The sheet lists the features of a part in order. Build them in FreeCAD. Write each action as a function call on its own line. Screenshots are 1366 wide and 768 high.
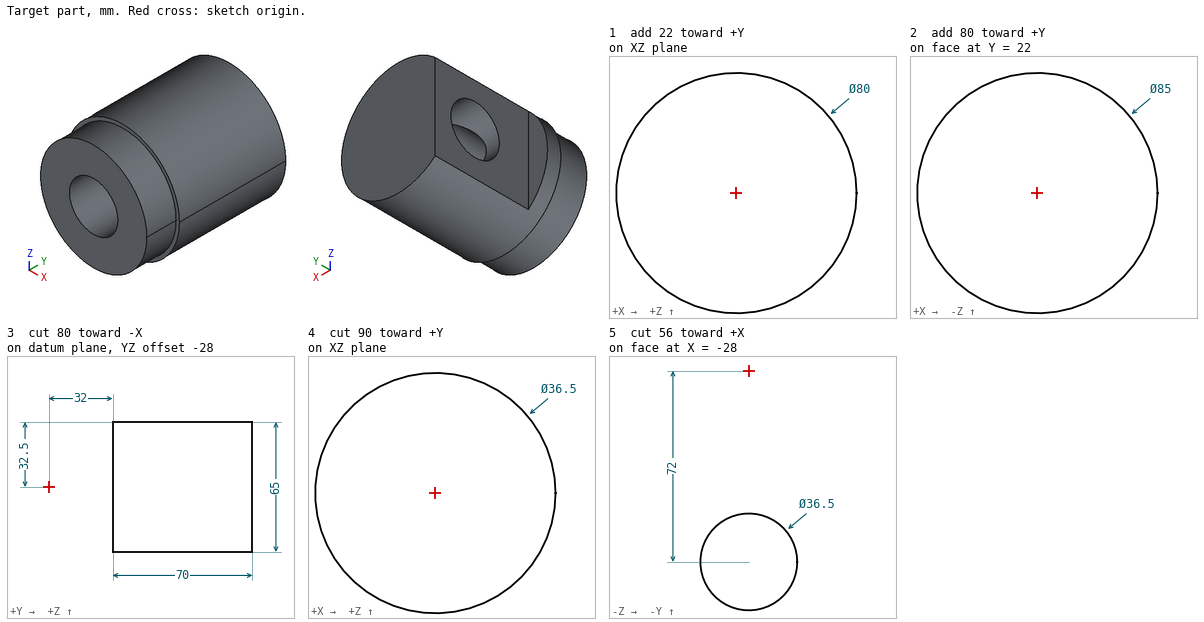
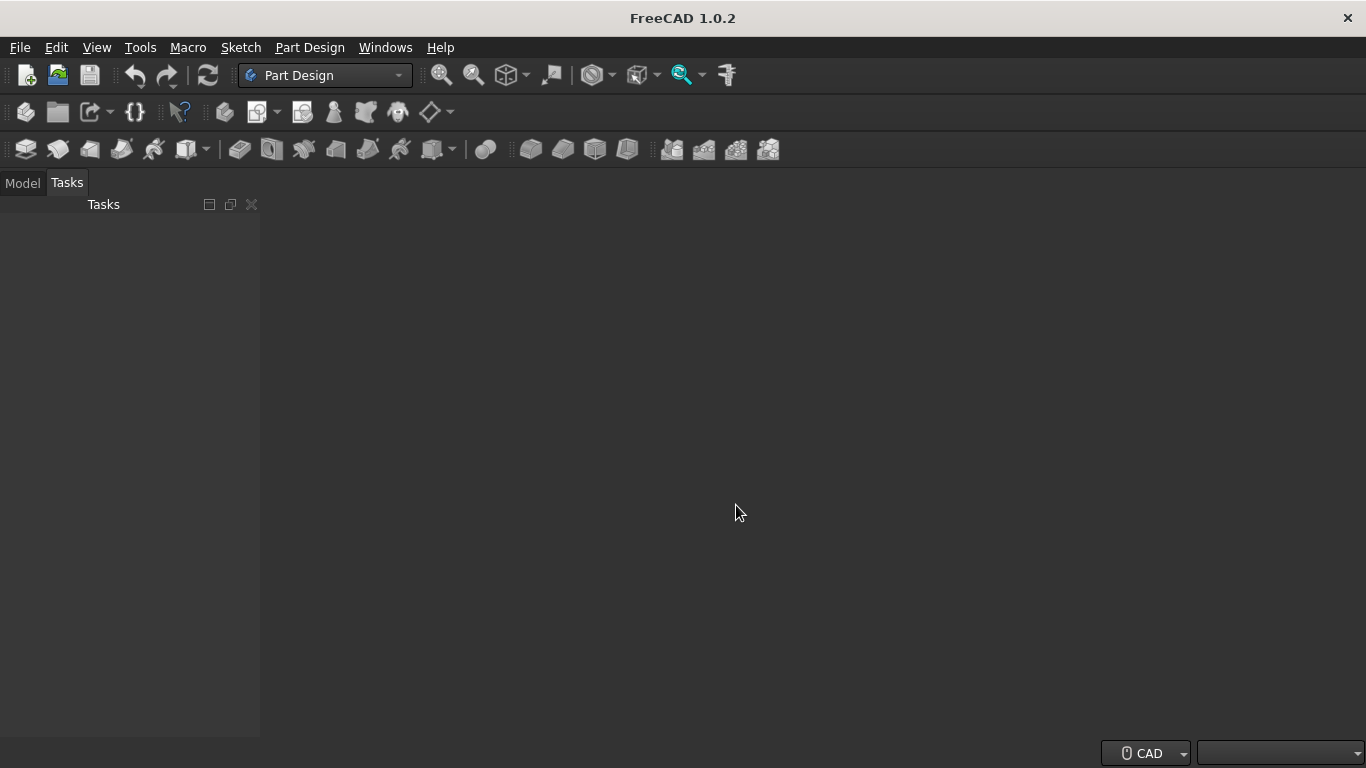
click(26, 76)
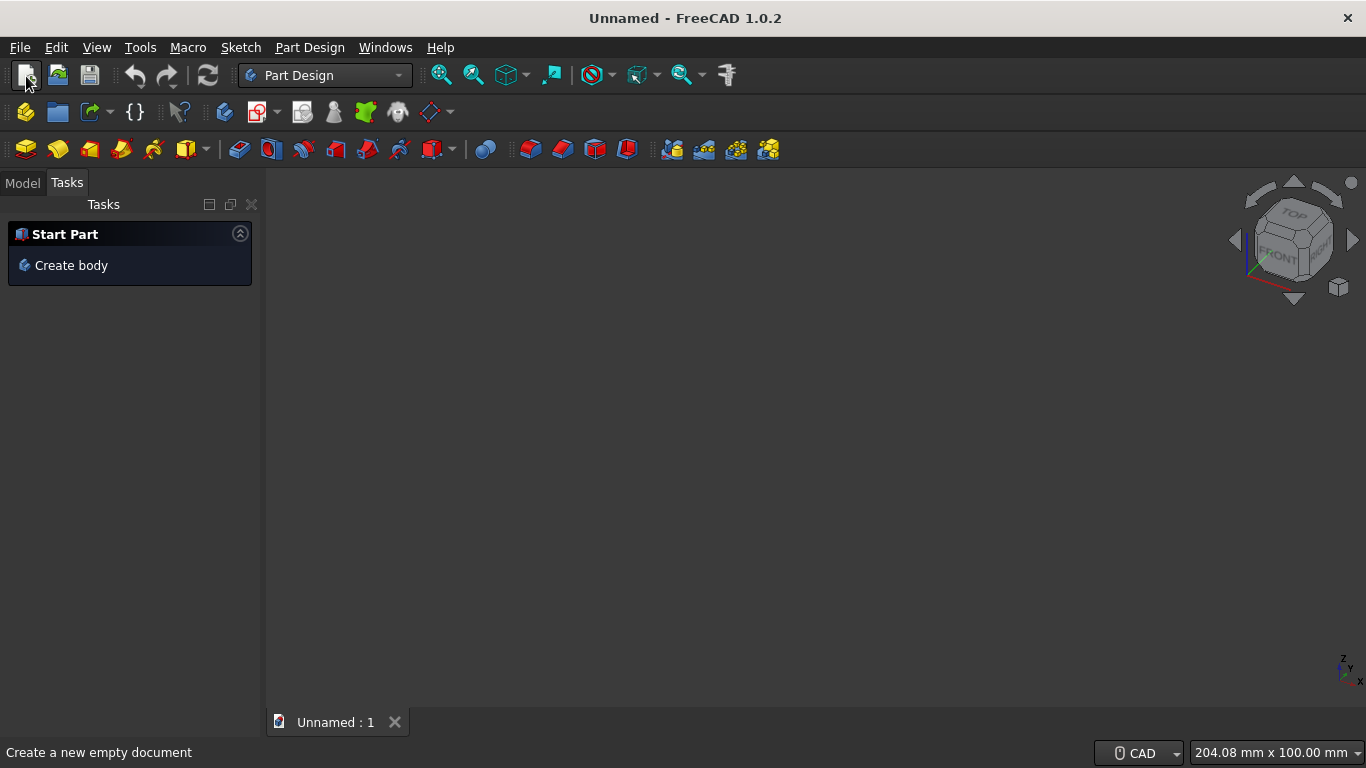
click(258, 112)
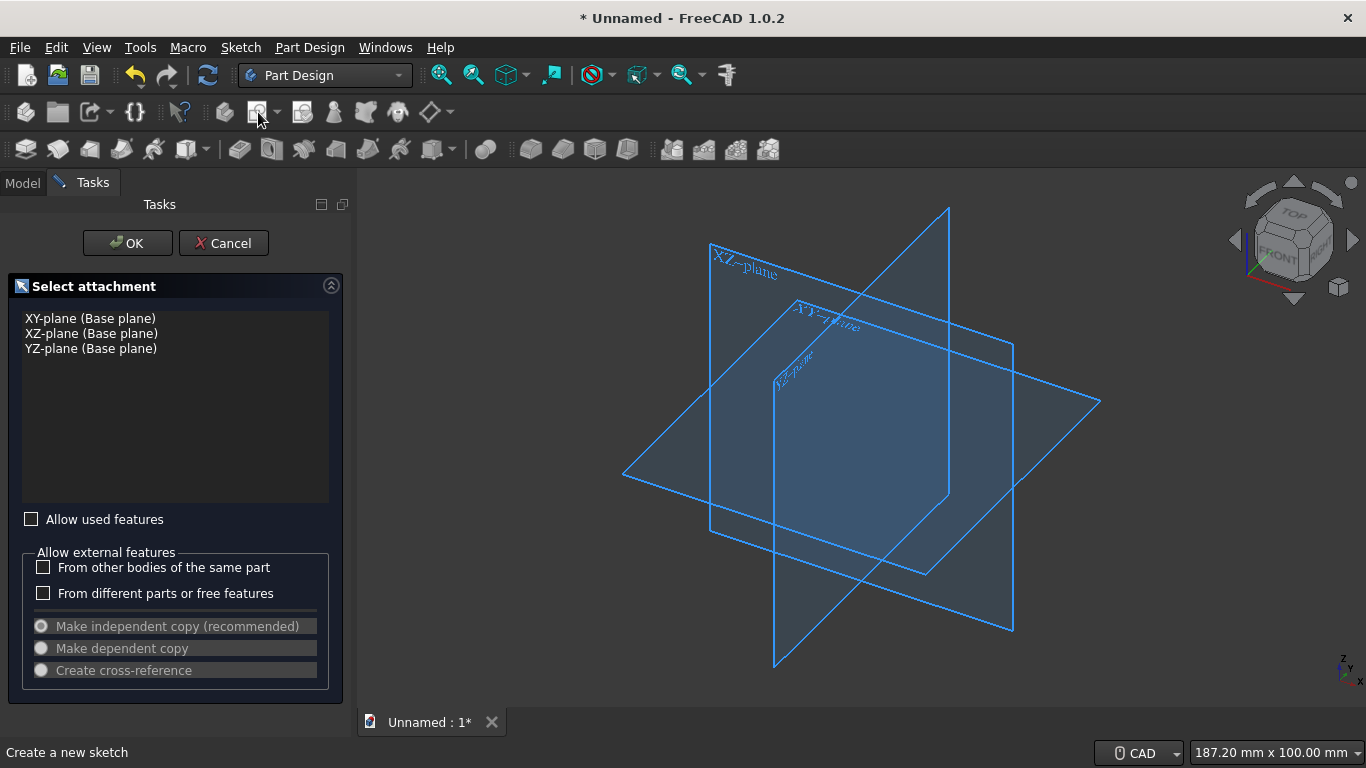
click(82, 334)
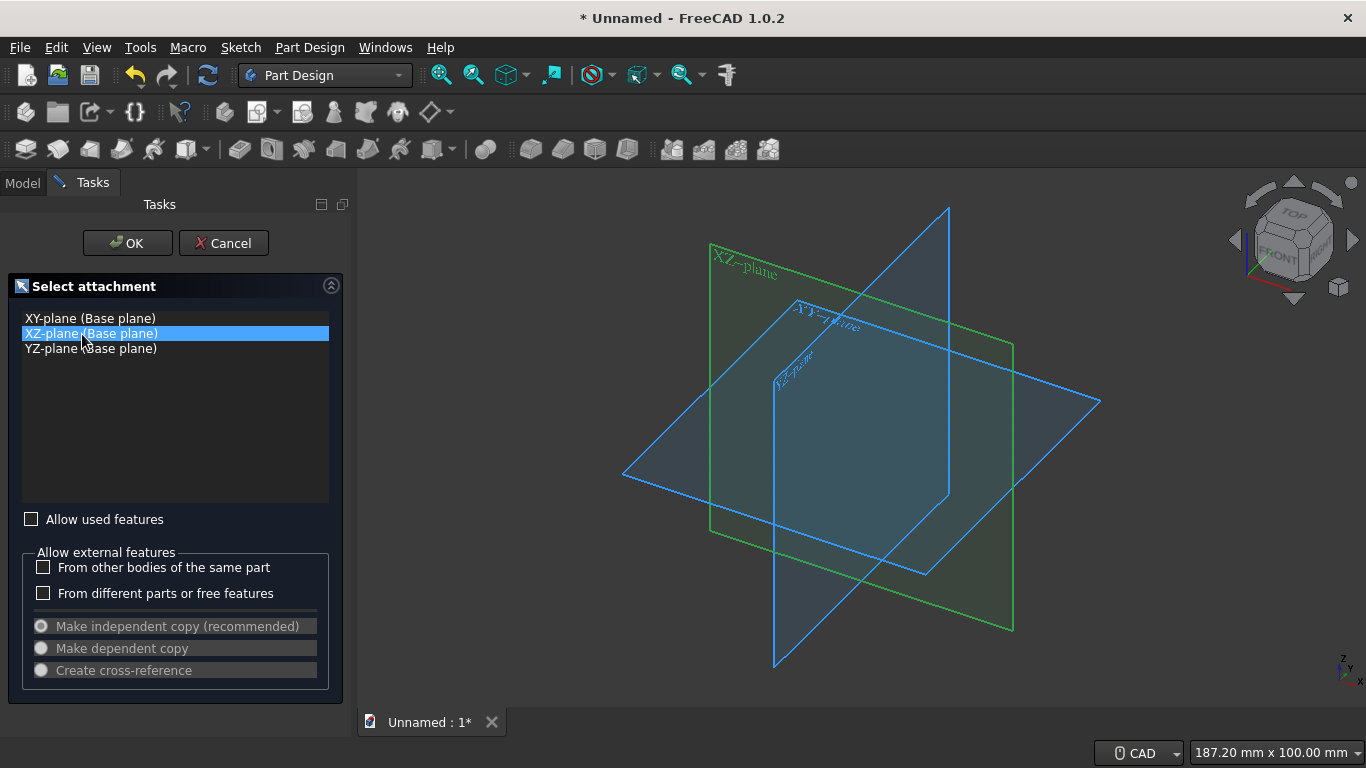
click(128, 243)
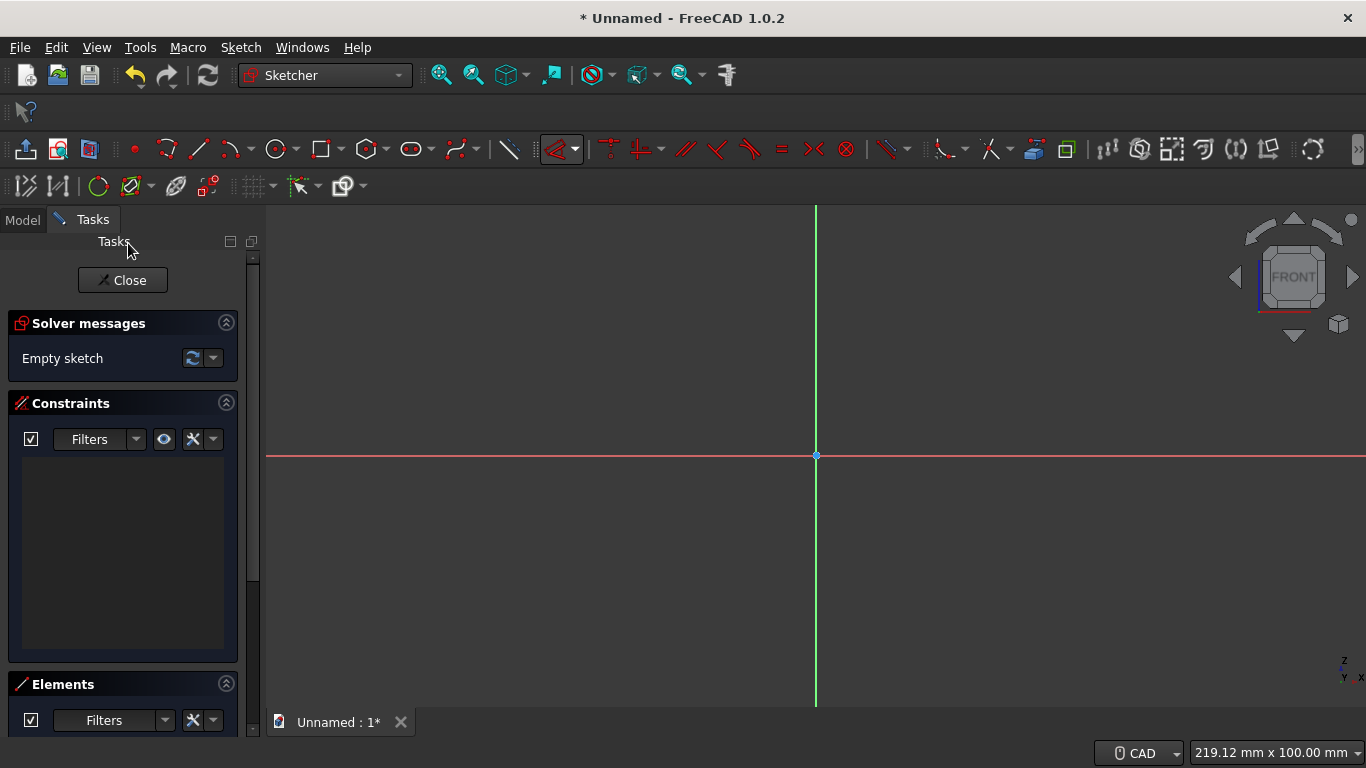
scroll(438, 456, down, 1)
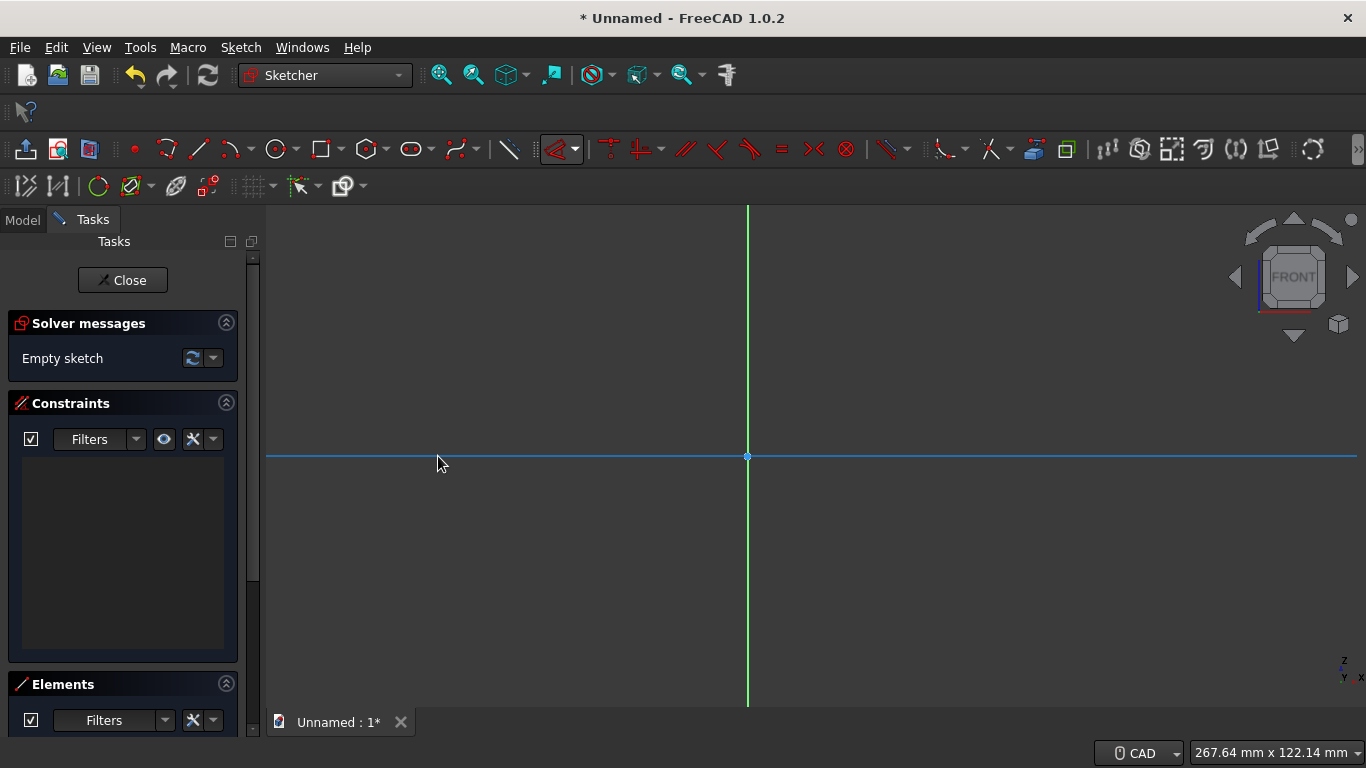
click(276, 150)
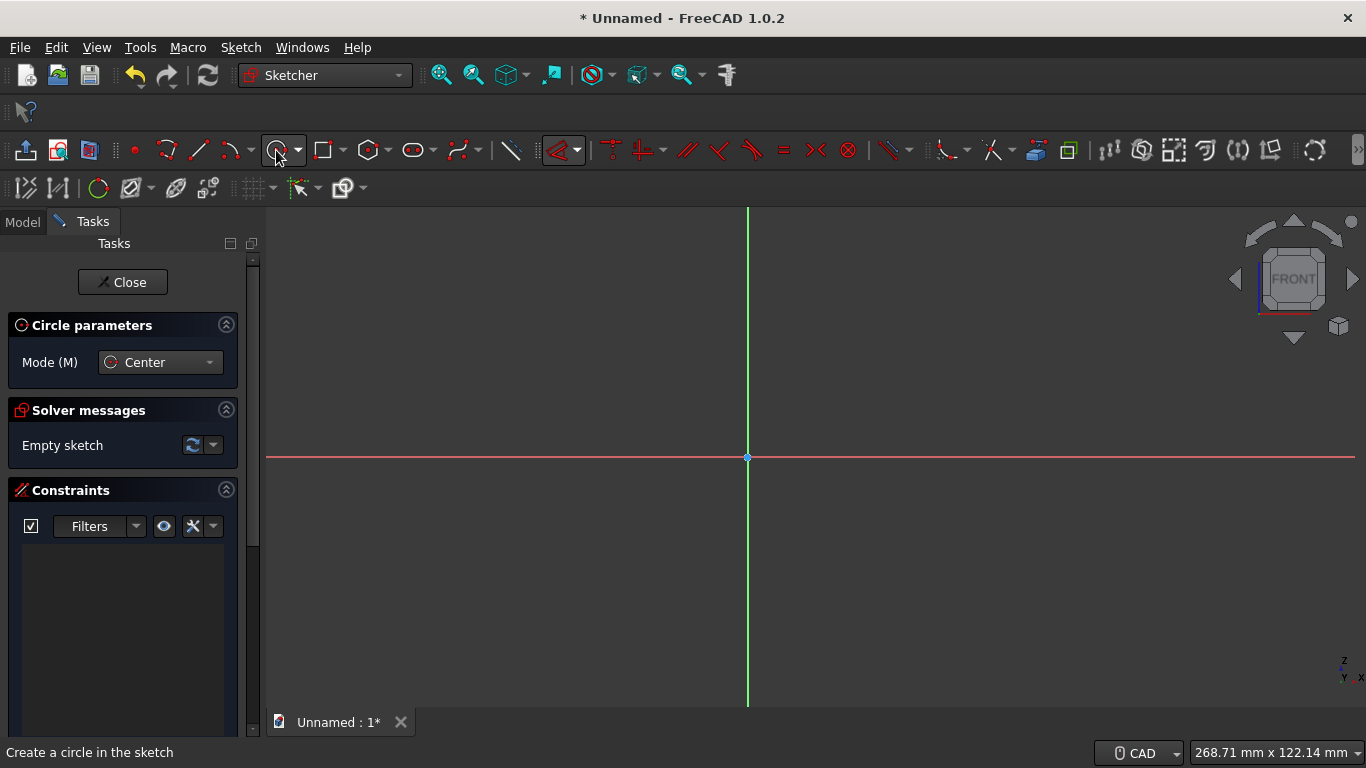
click(748, 457)
move(864, 341)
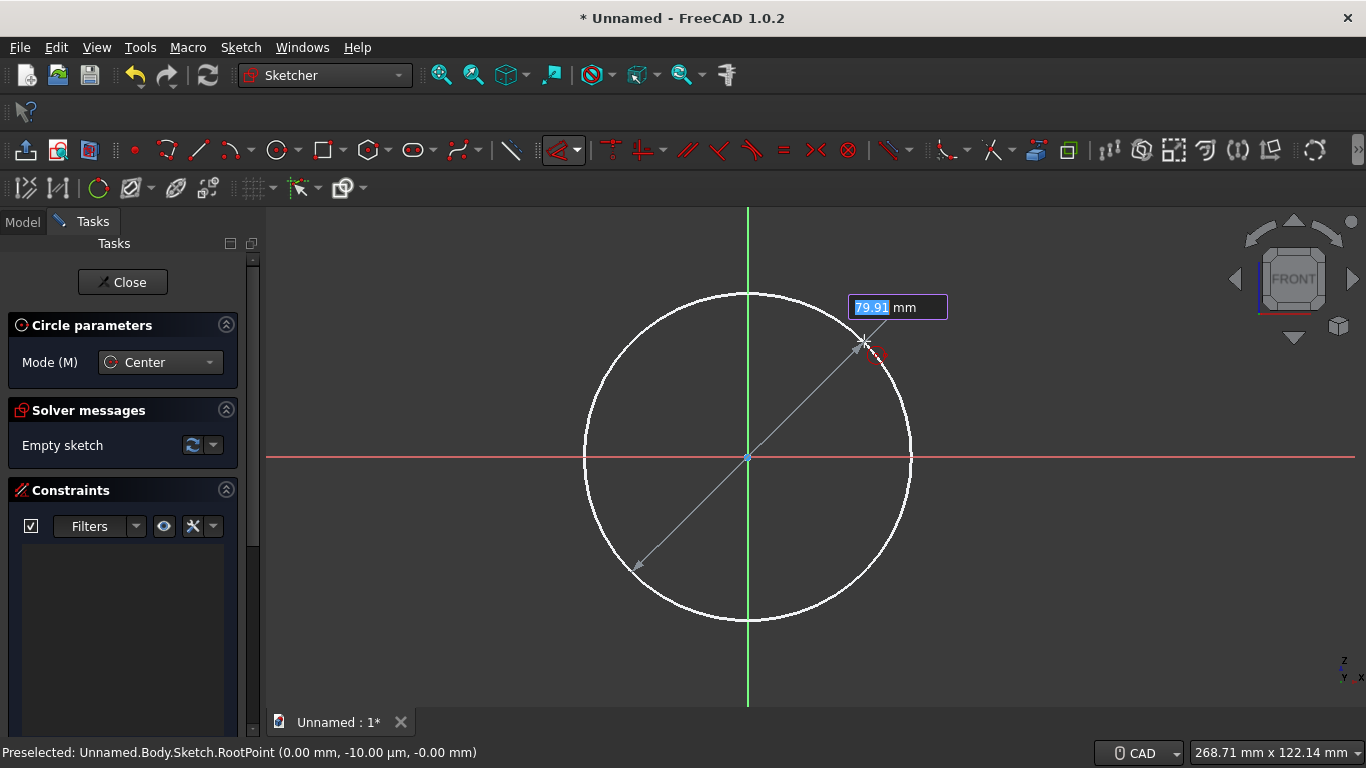
text(80)
key(Return)
key(Escape)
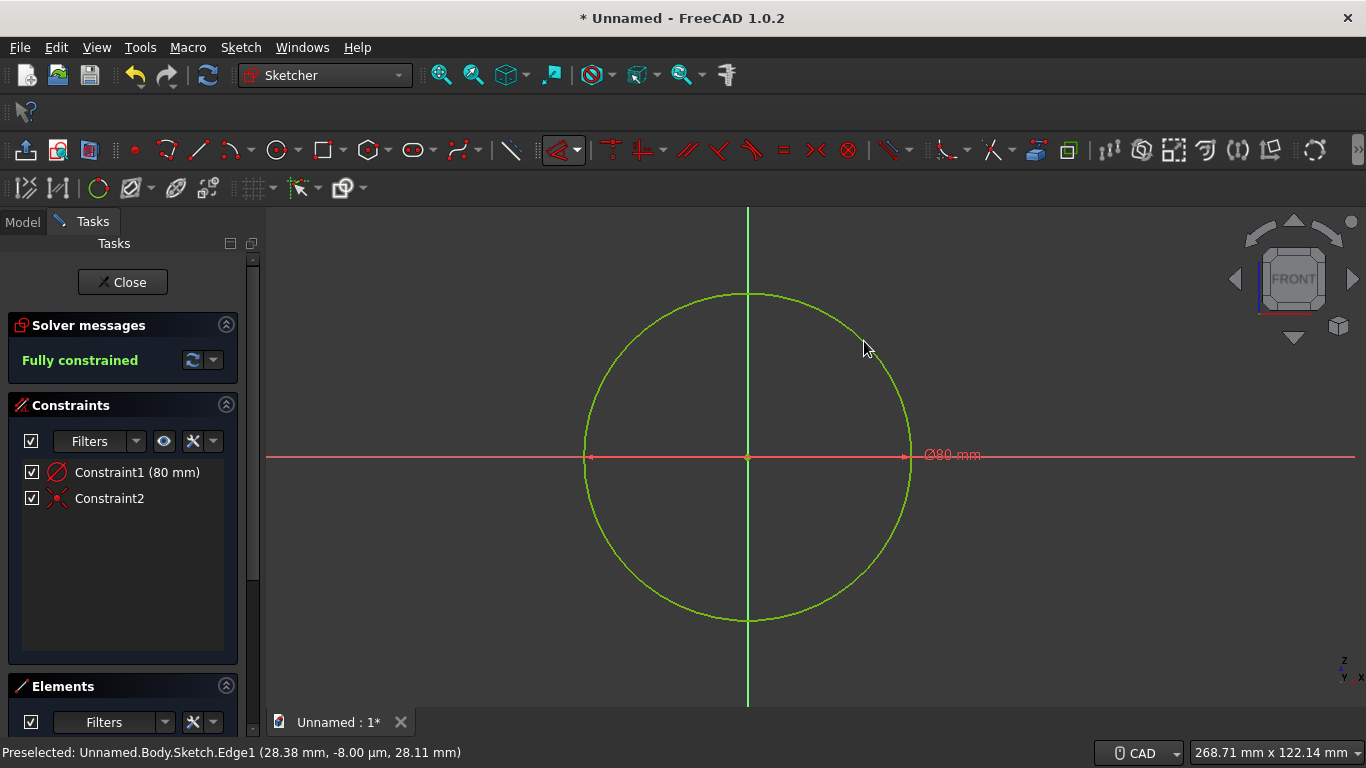
click(123, 282)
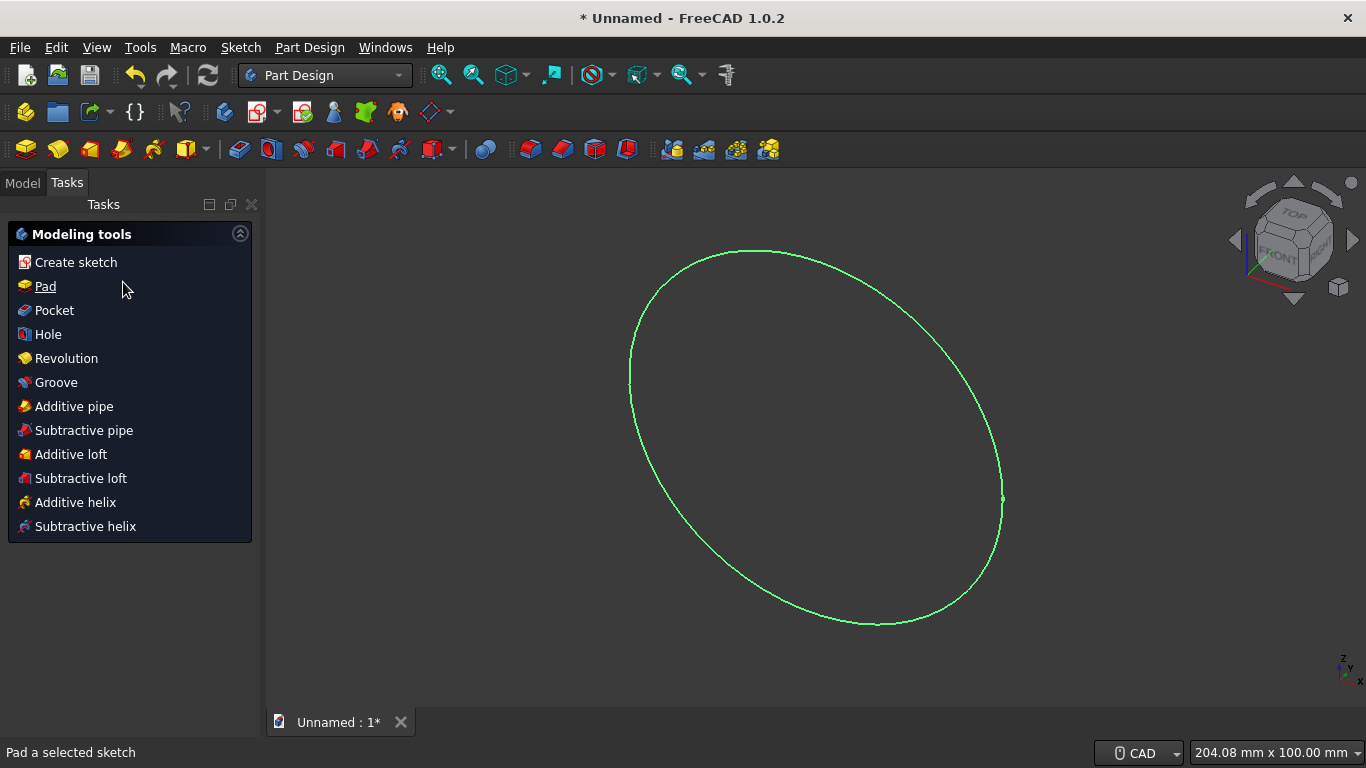
click(26, 150)